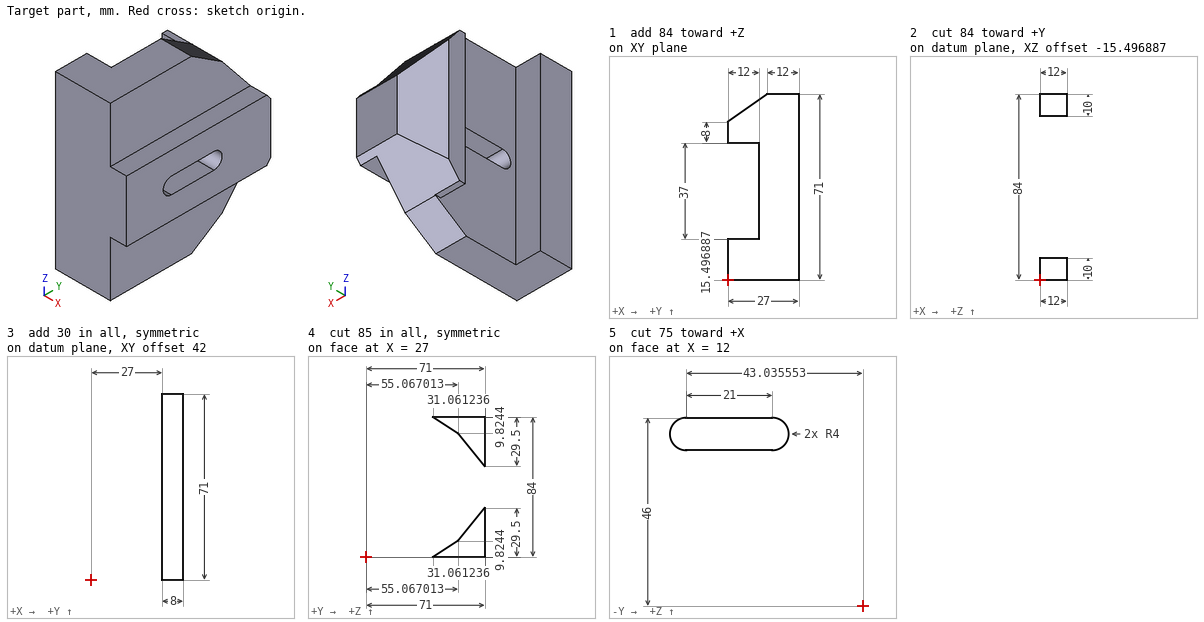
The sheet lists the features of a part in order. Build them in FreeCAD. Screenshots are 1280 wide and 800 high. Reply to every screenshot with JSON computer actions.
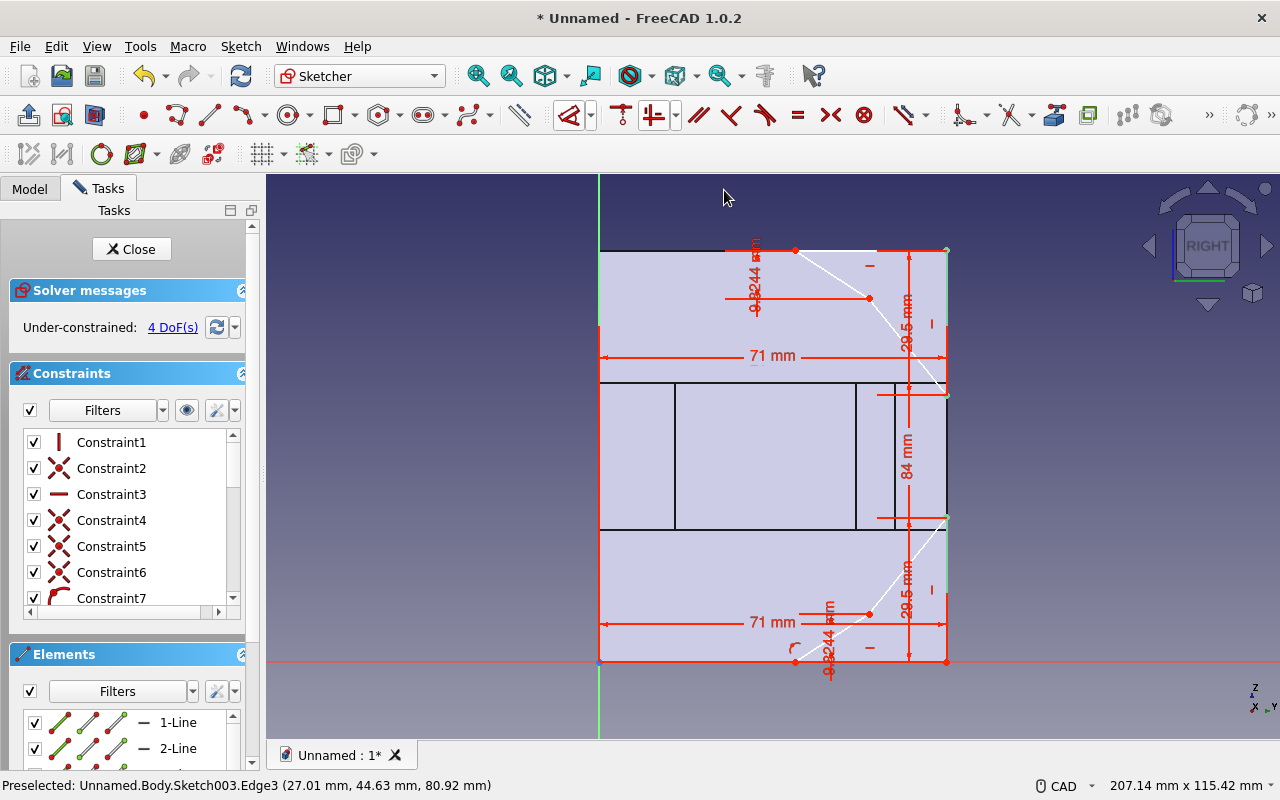
{"action": "left_click", "coordinate": [901, 251]}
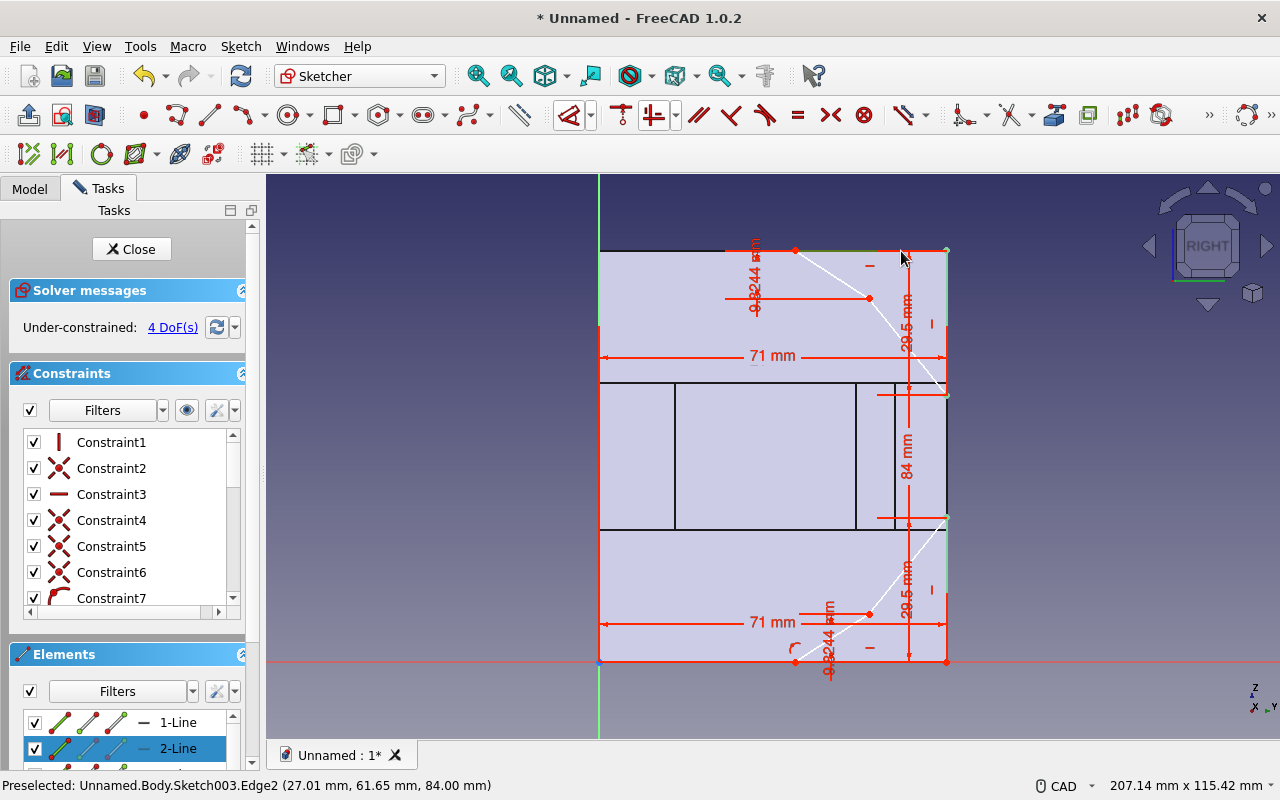
{"action": "left_click", "coordinate": [590, 116]}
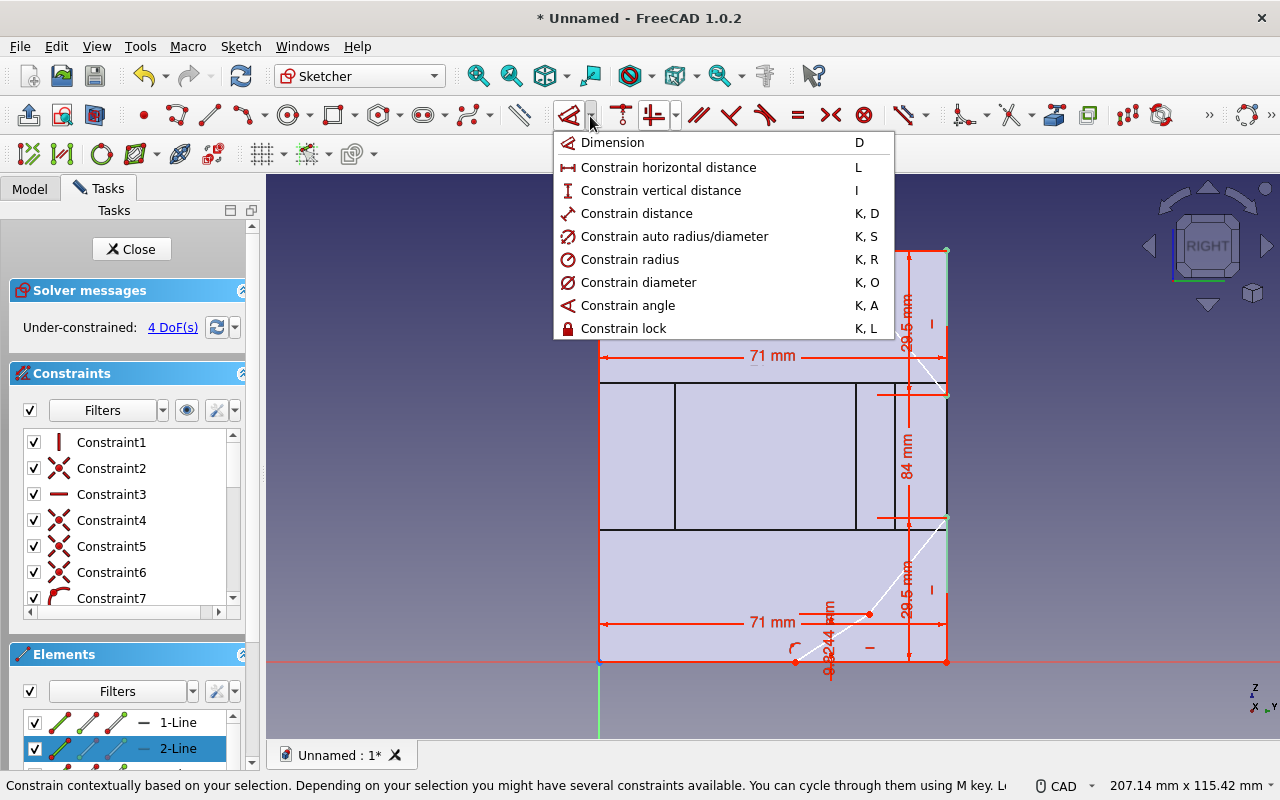
{"action": "left_click", "coordinate": [724, 168]}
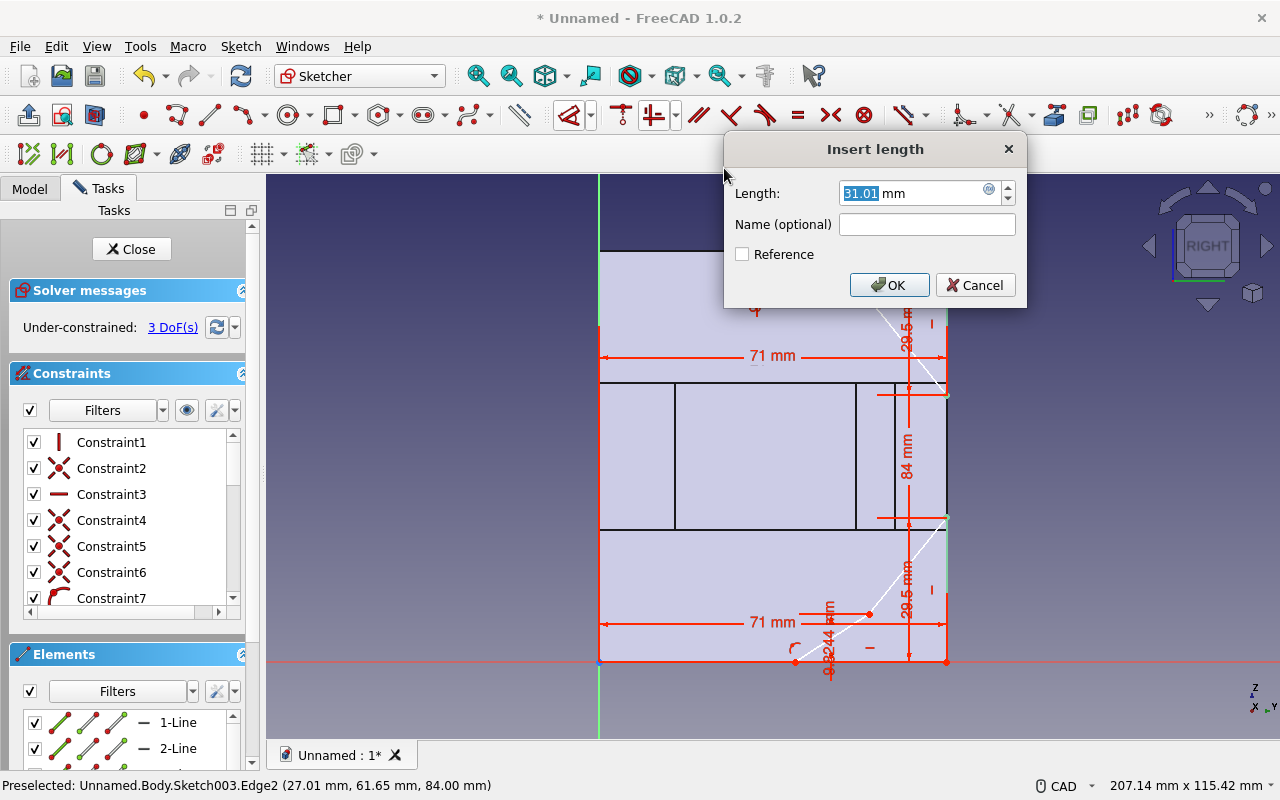
{"action": "type", "text": "31.061236"}
{"action": "key", "text": "Return"}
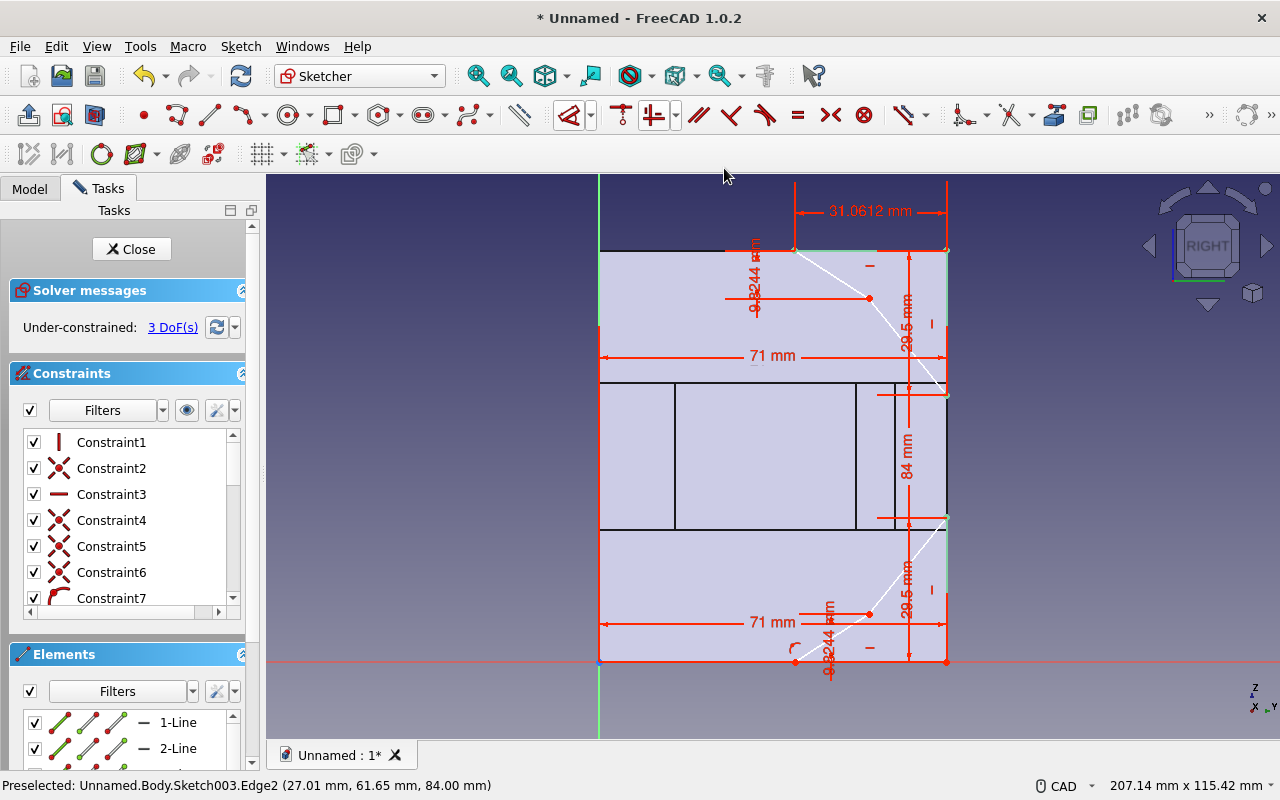
{"action": "left_click", "coordinate": [841, 662]}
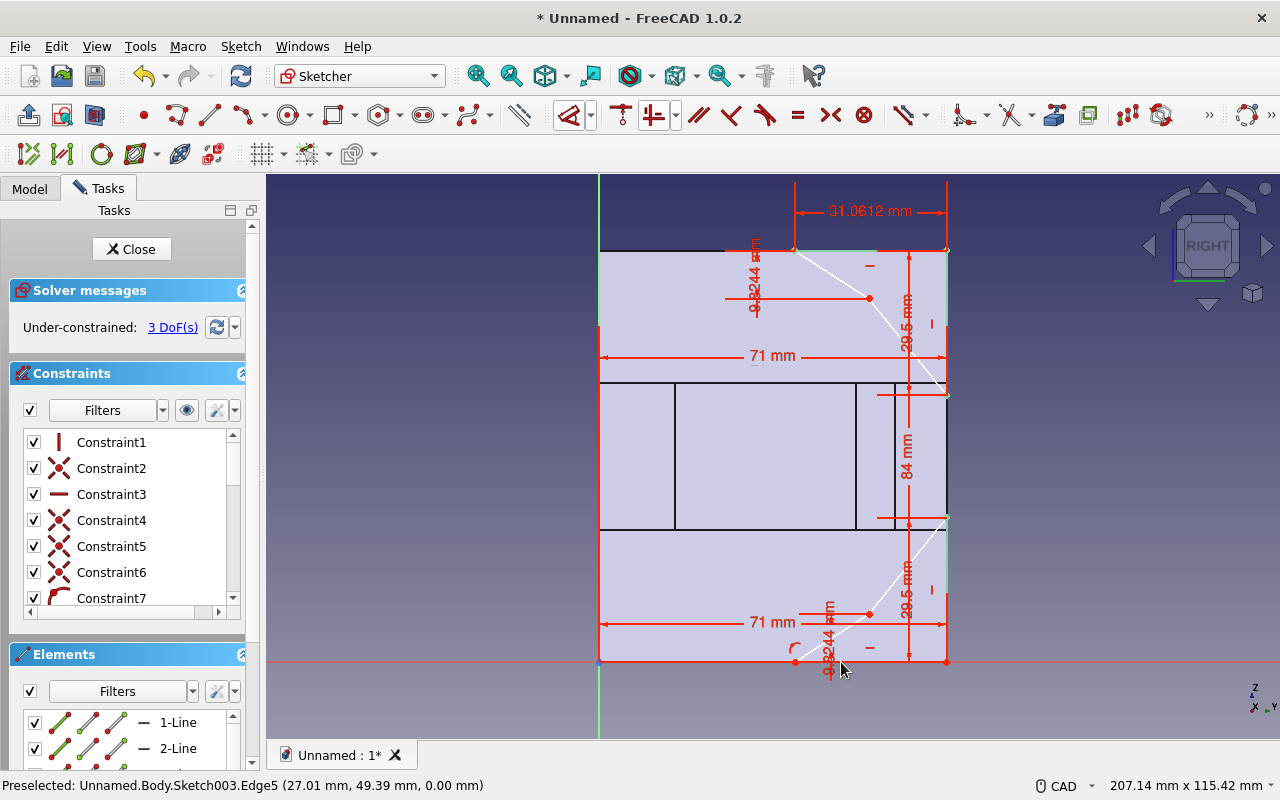
{"action": "key", "text": "l"}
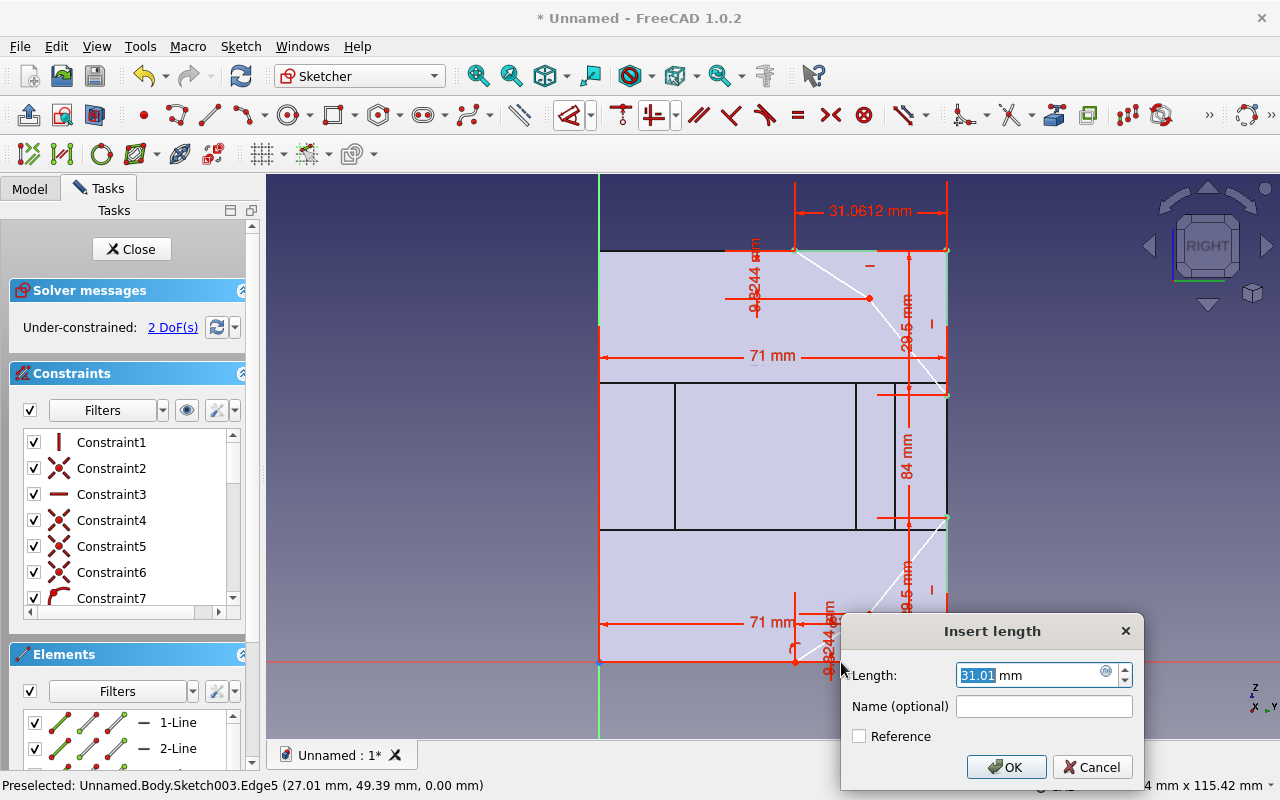
{"action": "type", "text": "31.061236"}
{"action": "key", "text": "Return"}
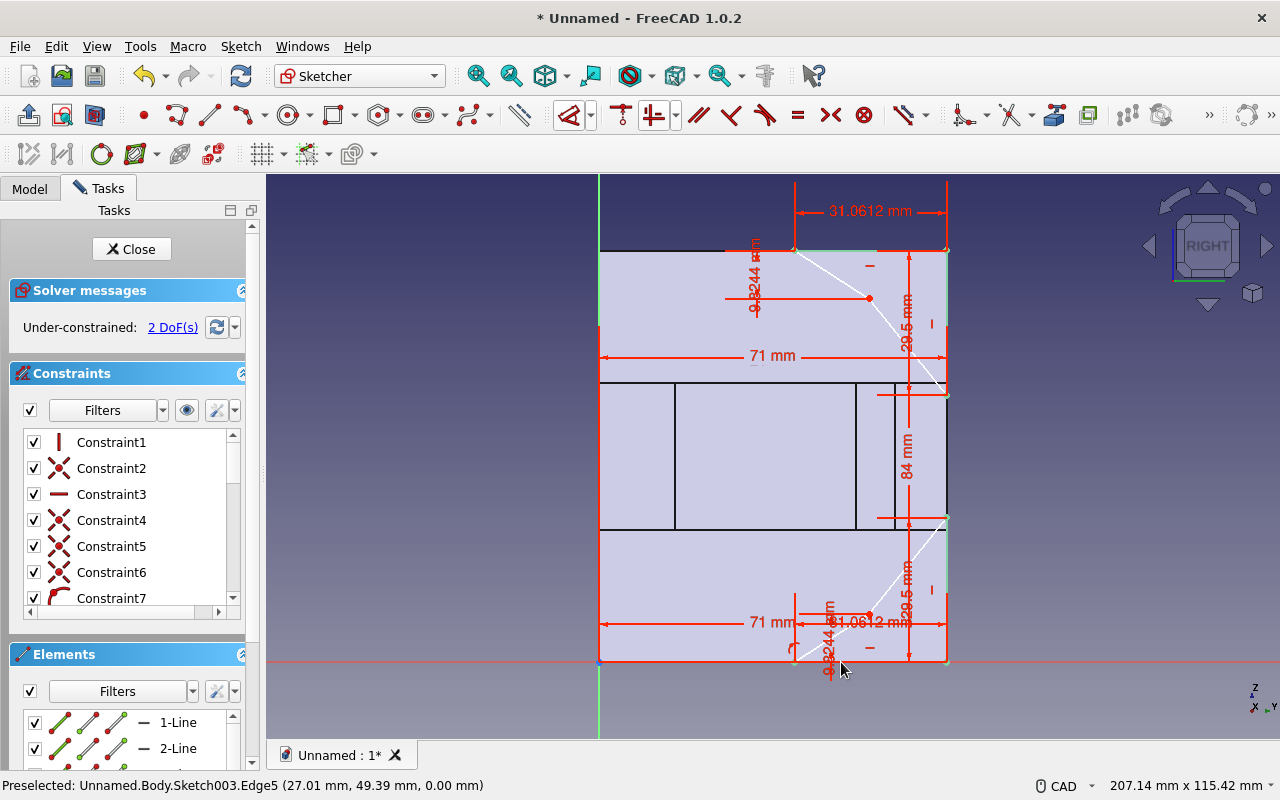
{"action": "left_click", "coordinate": [869, 299]}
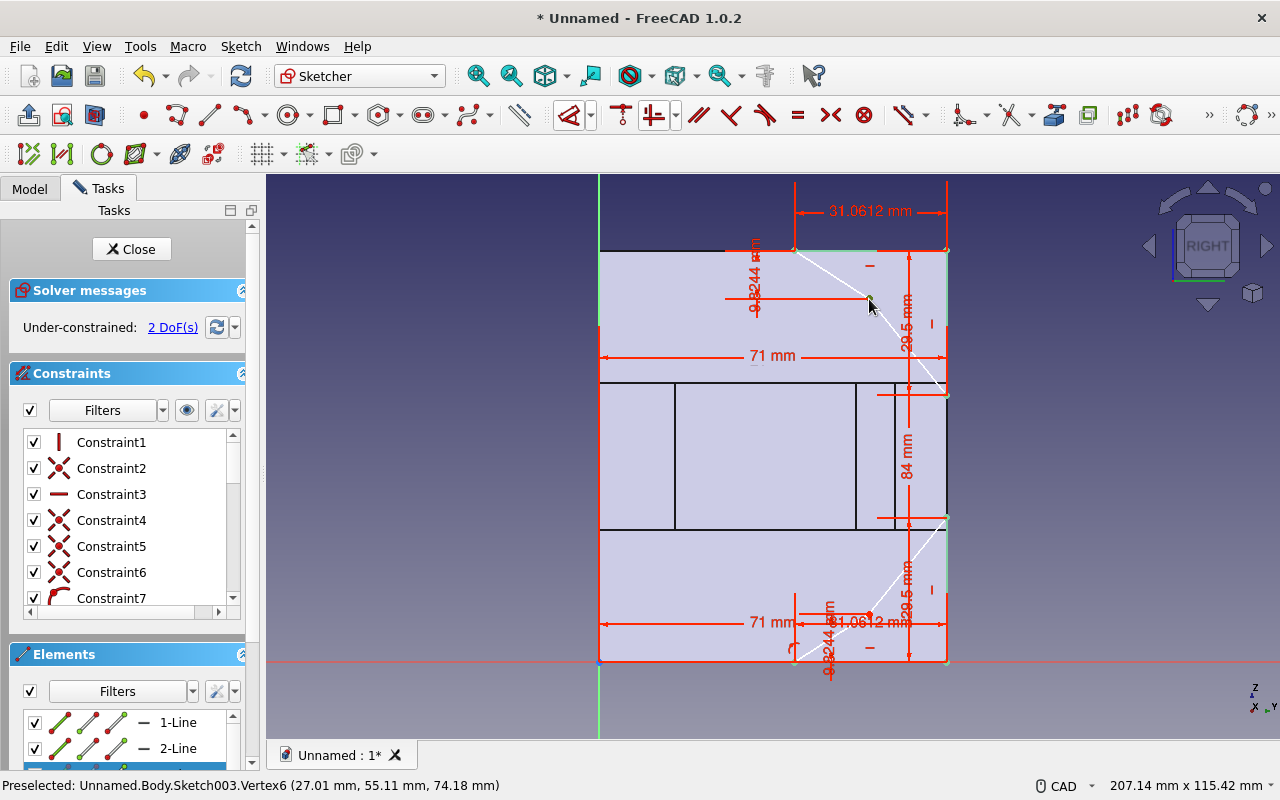
{"action": "left_click", "coordinate": [590, 116]}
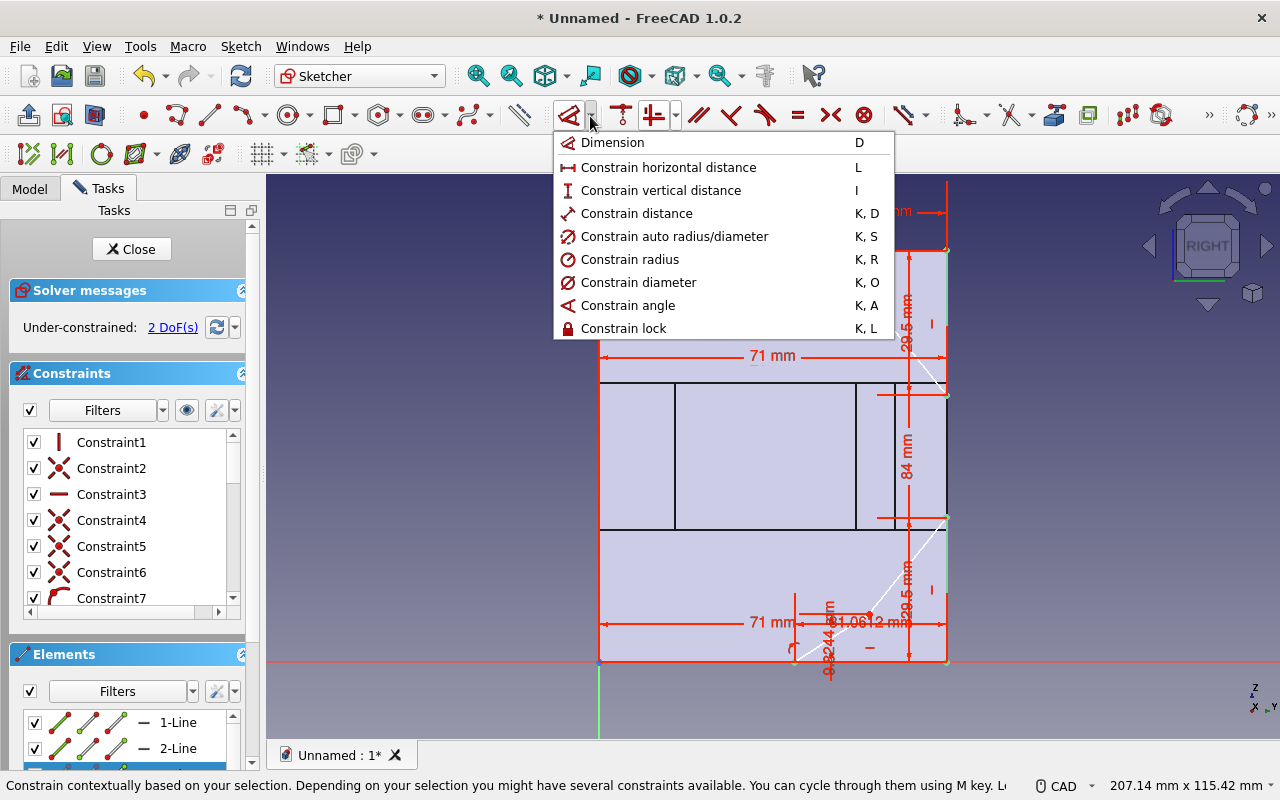
{"action": "left_click", "coordinate": [724, 168]}